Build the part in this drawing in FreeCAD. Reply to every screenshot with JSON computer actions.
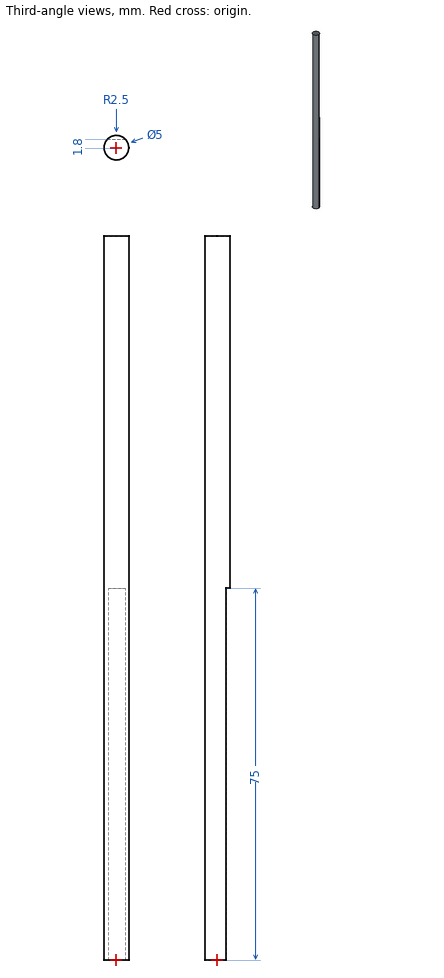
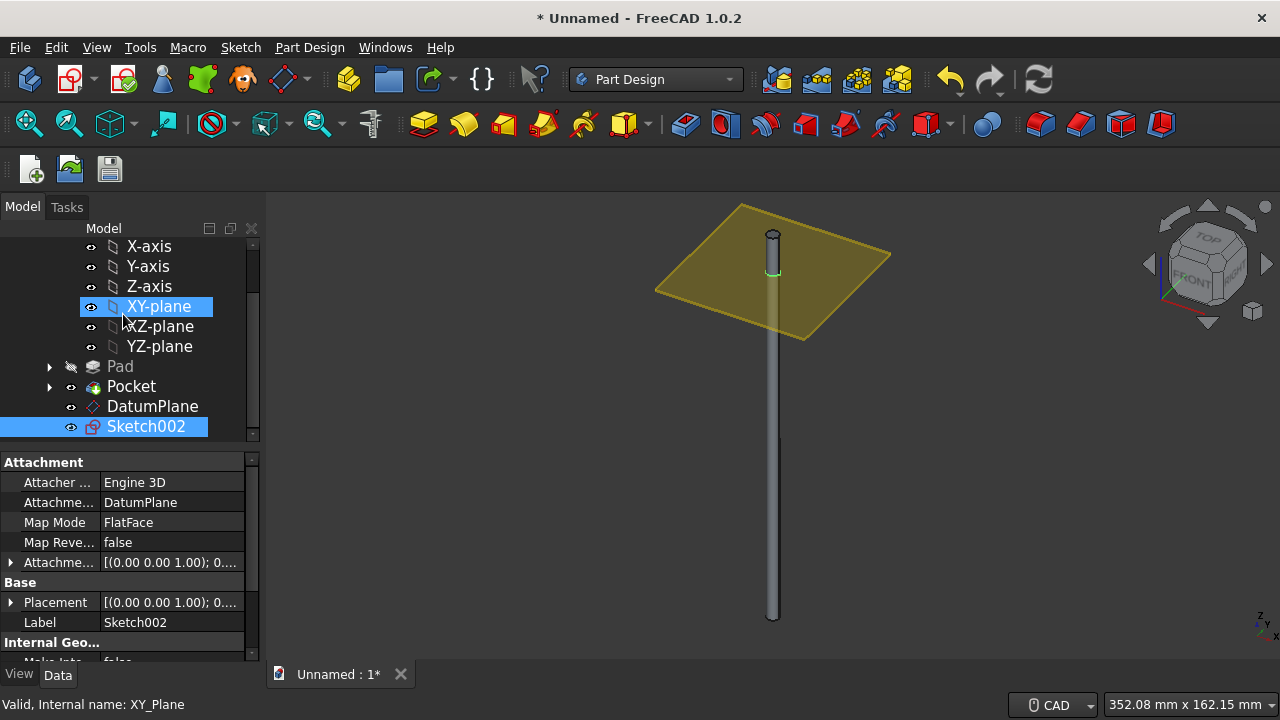
{"action": "left_click", "coordinate": [686, 124]}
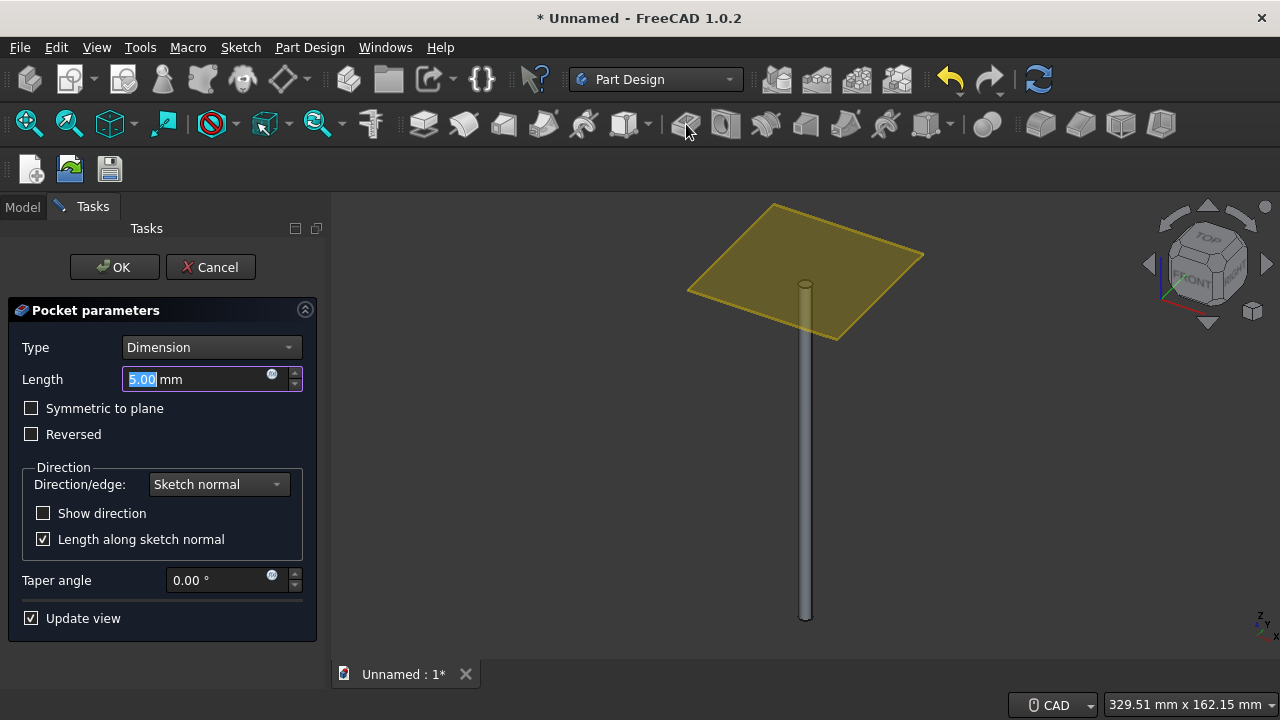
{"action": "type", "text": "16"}
{"action": "key", "text": "Tab"}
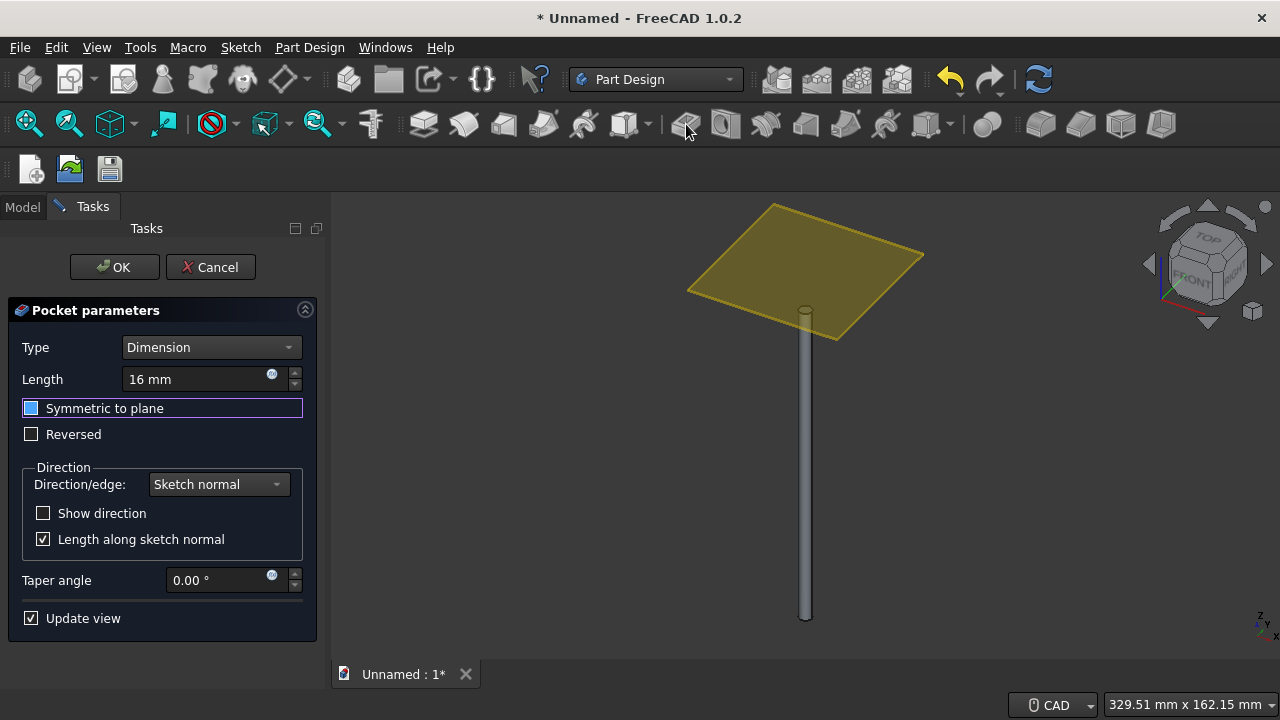
{"action": "left_click", "coordinate": [30, 434]}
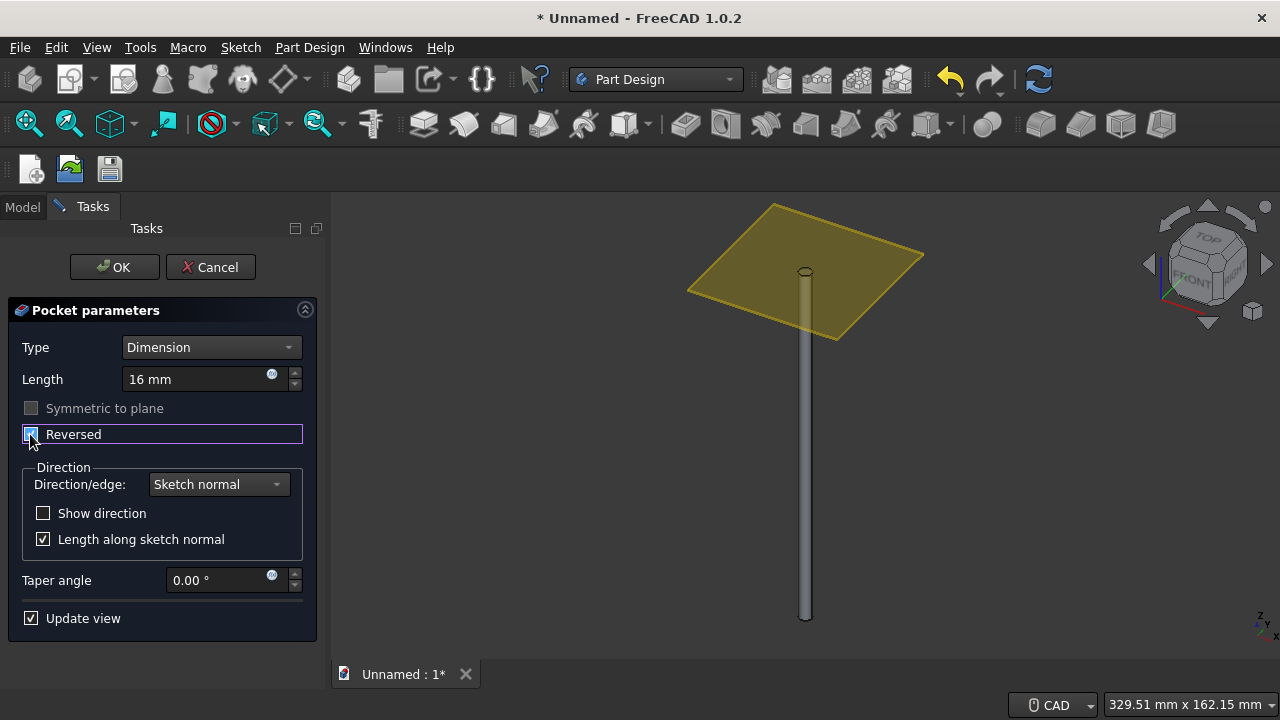
{"action": "left_click", "coordinate": [115, 267]}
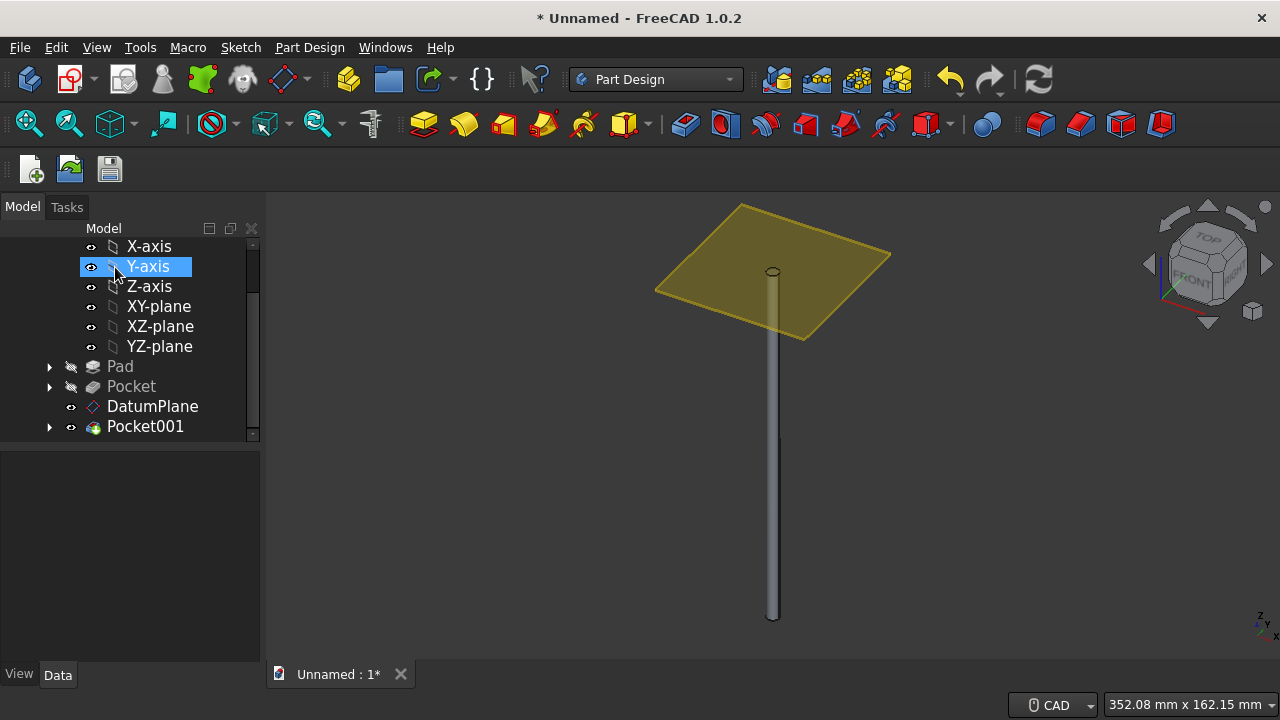
{"action": "left_click", "coordinate": [116, 407]}
{"action": "key", "text": "space"}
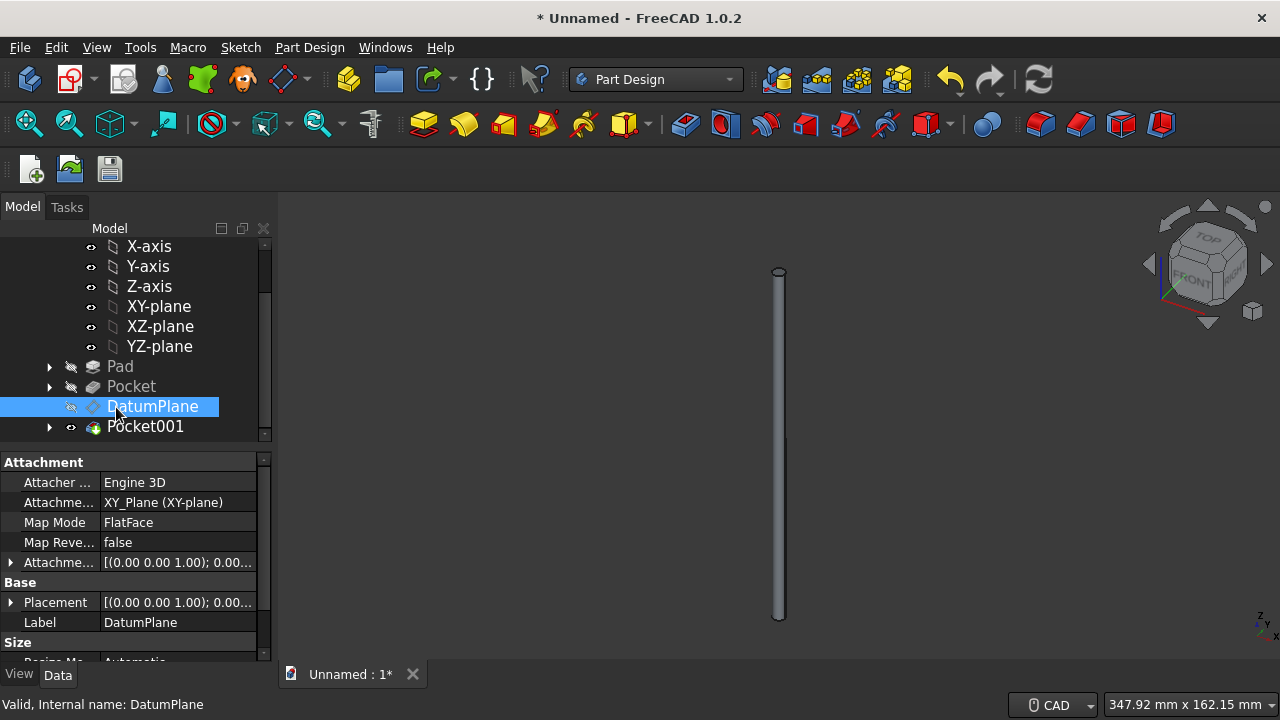
{"action": "key", "text": "0"}